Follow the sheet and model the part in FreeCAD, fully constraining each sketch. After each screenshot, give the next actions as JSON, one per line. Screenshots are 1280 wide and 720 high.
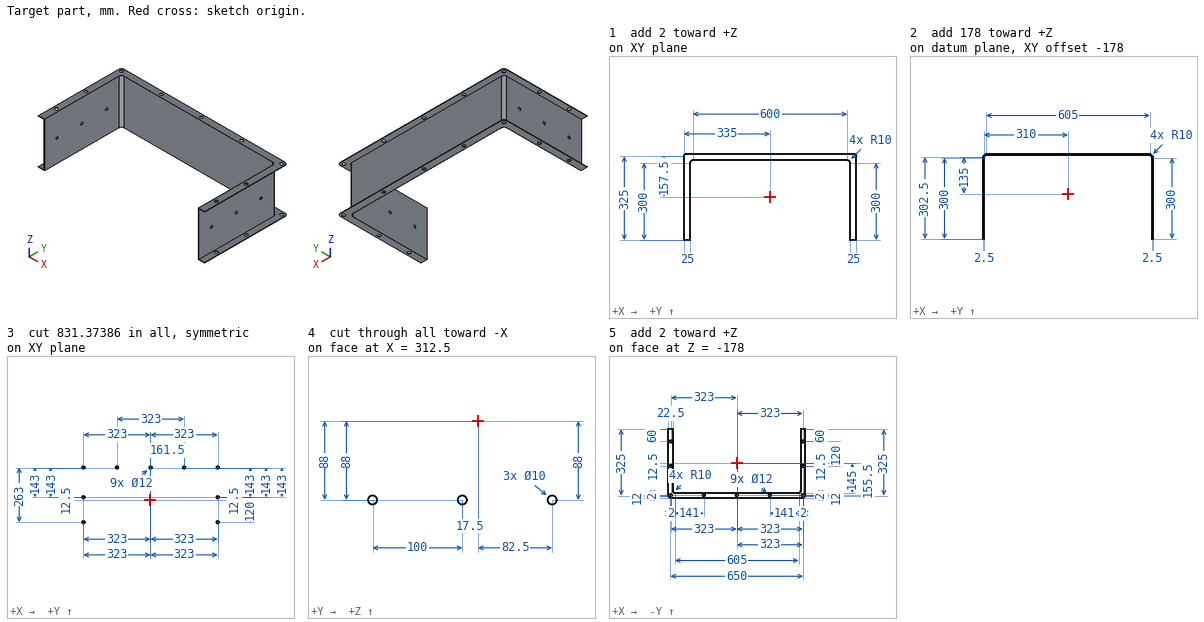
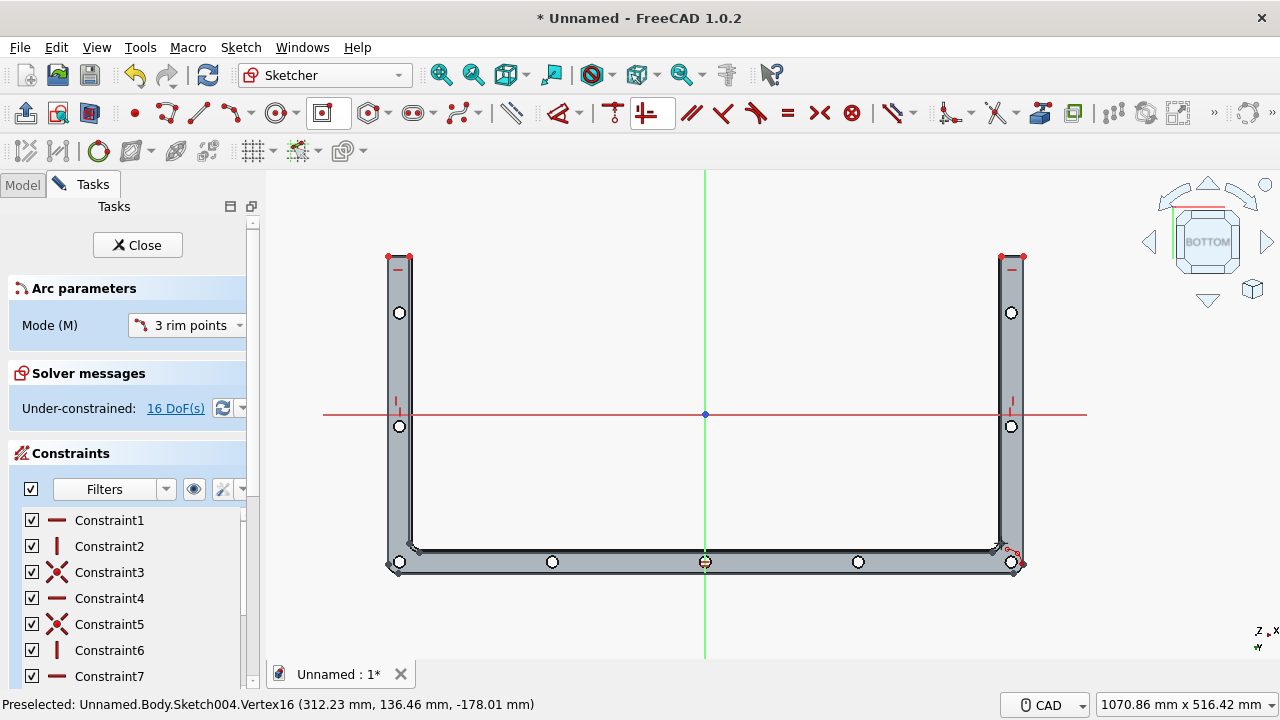
{"action": "left_click", "coordinate": [419, 553]}
{"action": "left_click", "coordinate": [409, 544]}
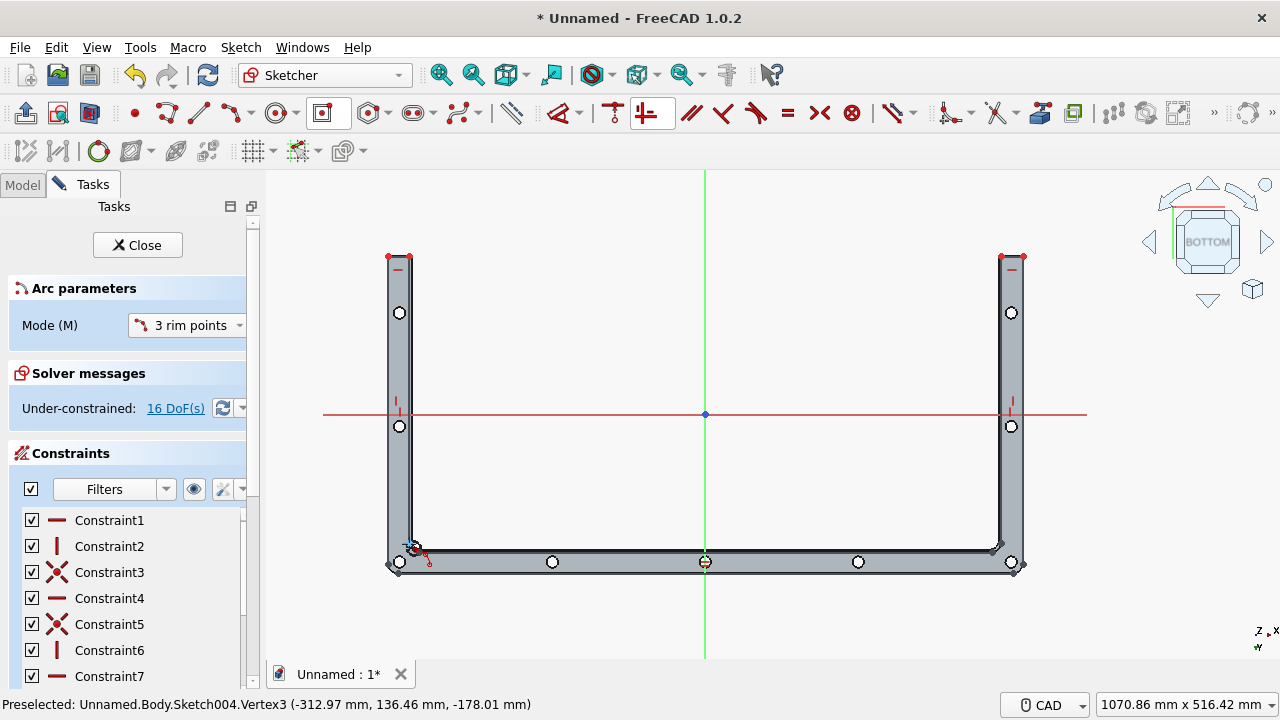
{"action": "scroll", "coordinate": [412, 549], "scroll_direction": "up", "scroll_amount": 9}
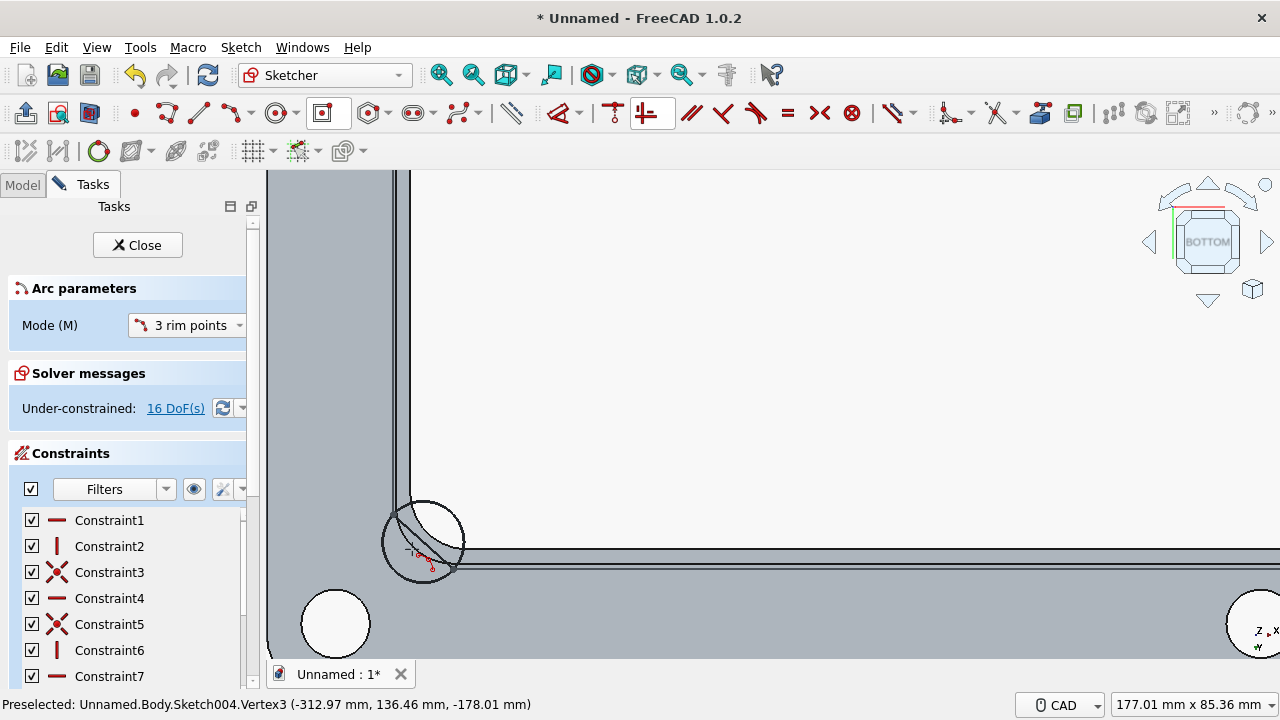
{"action": "left_click", "coordinate": [413, 547]}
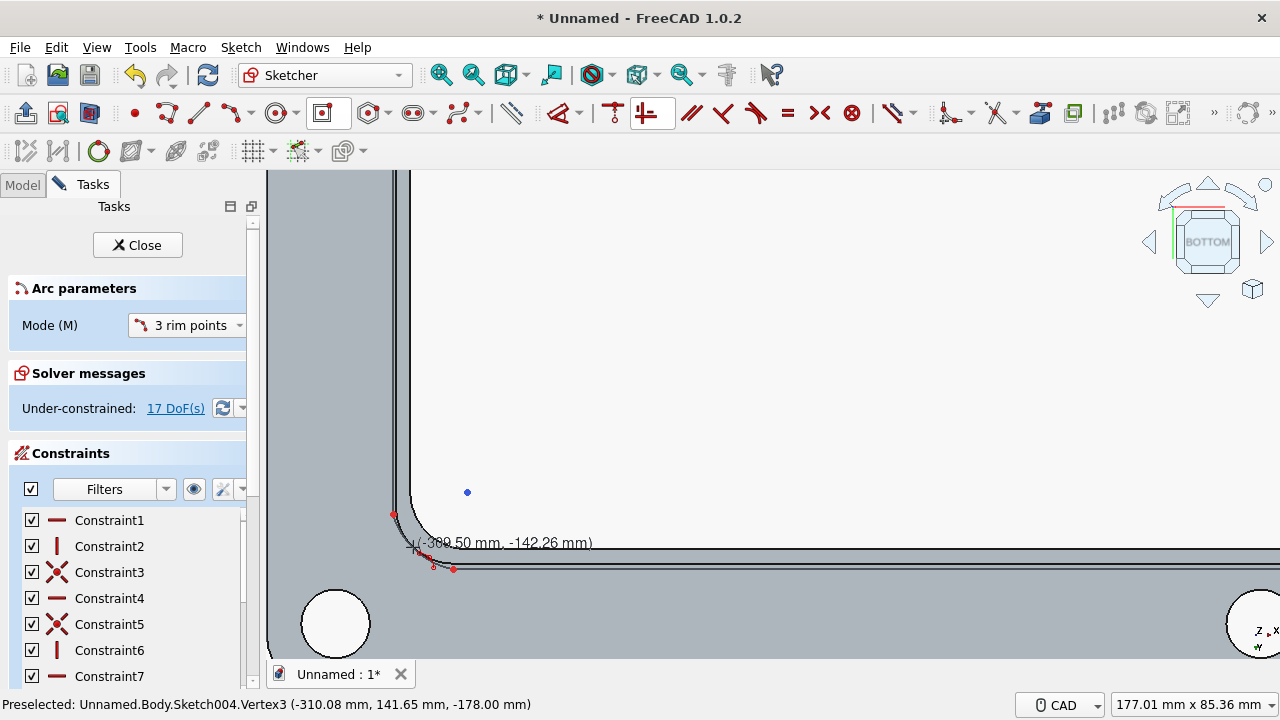
{"action": "scroll", "coordinate": [411, 549], "scroll_direction": "down", "scroll_amount": 9}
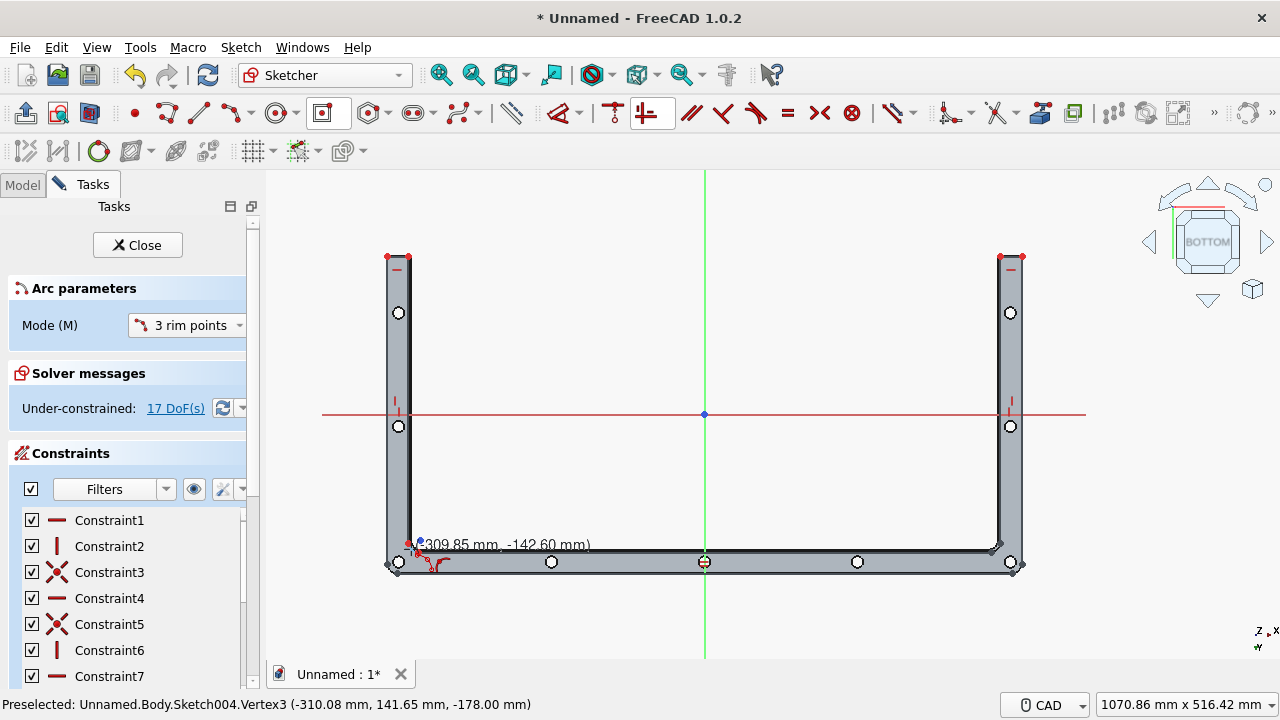
{"action": "left_click", "coordinate": [387, 565]}
{"action": "left_click", "coordinate": [397, 574]}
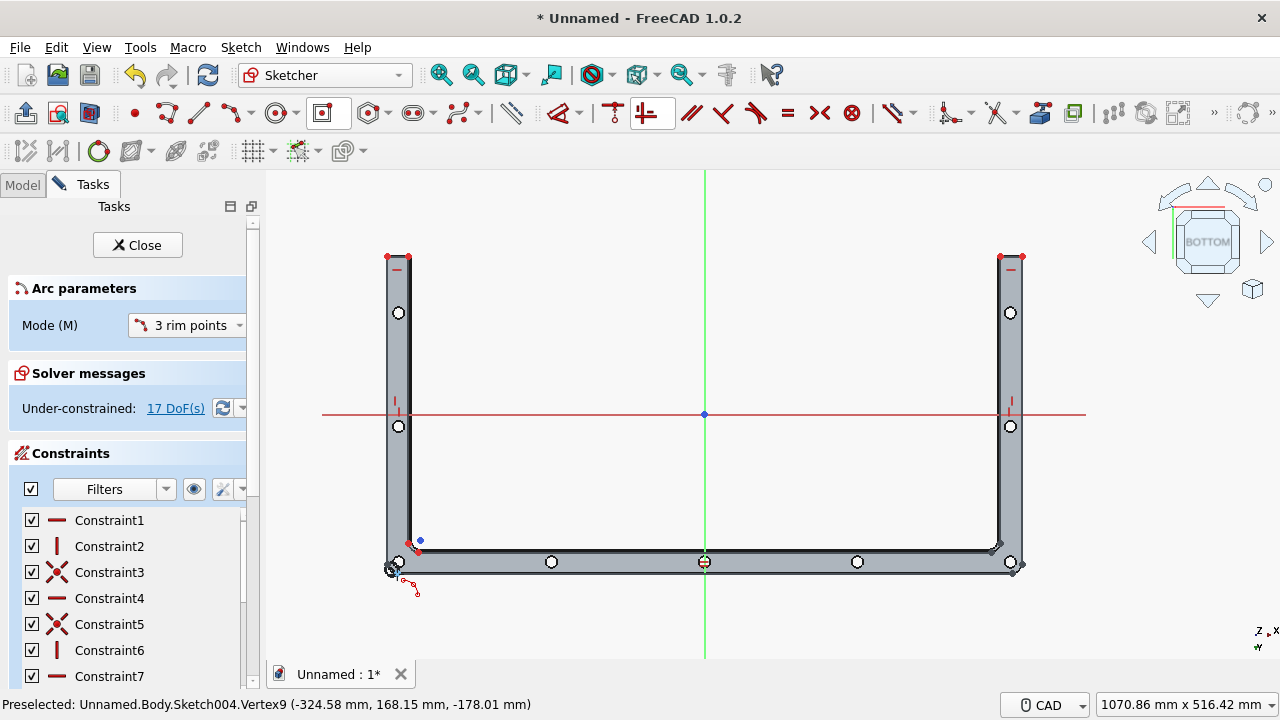
{"action": "scroll", "coordinate": [390, 571], "scroll_direction": "up", "scroll_amount": 9}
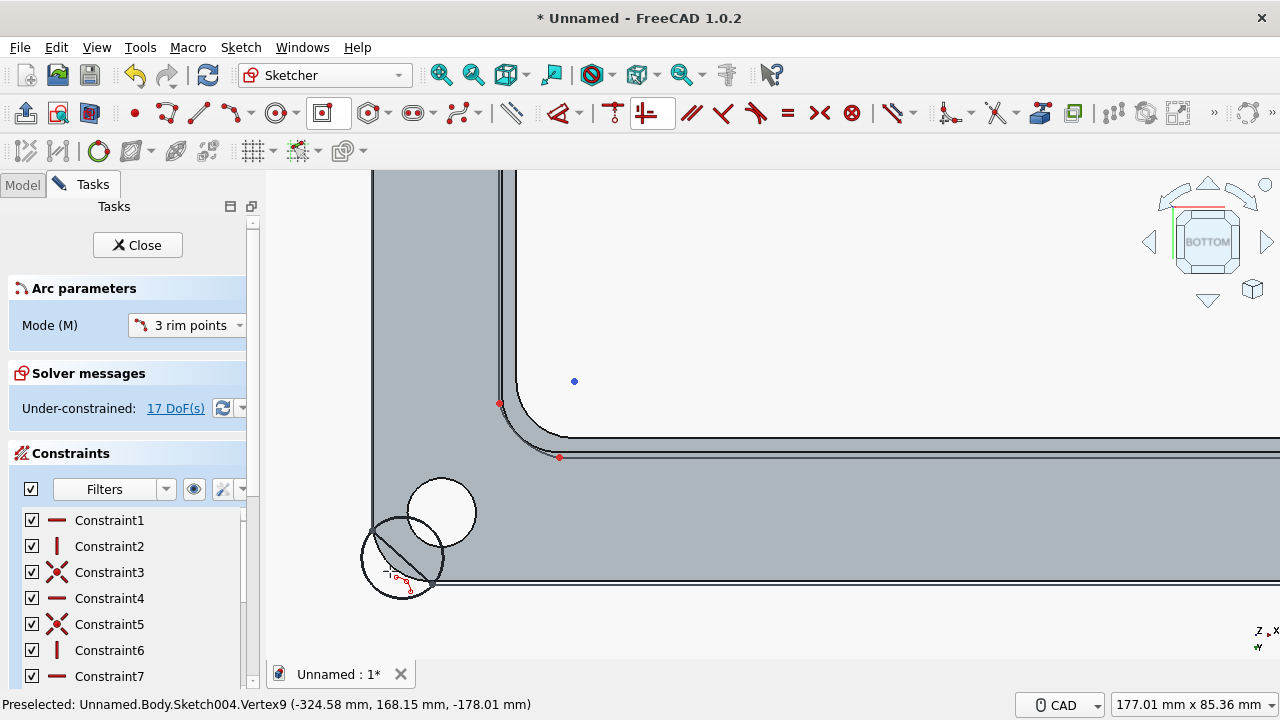
{"action": "left_click", "coordinate": [390, 565]}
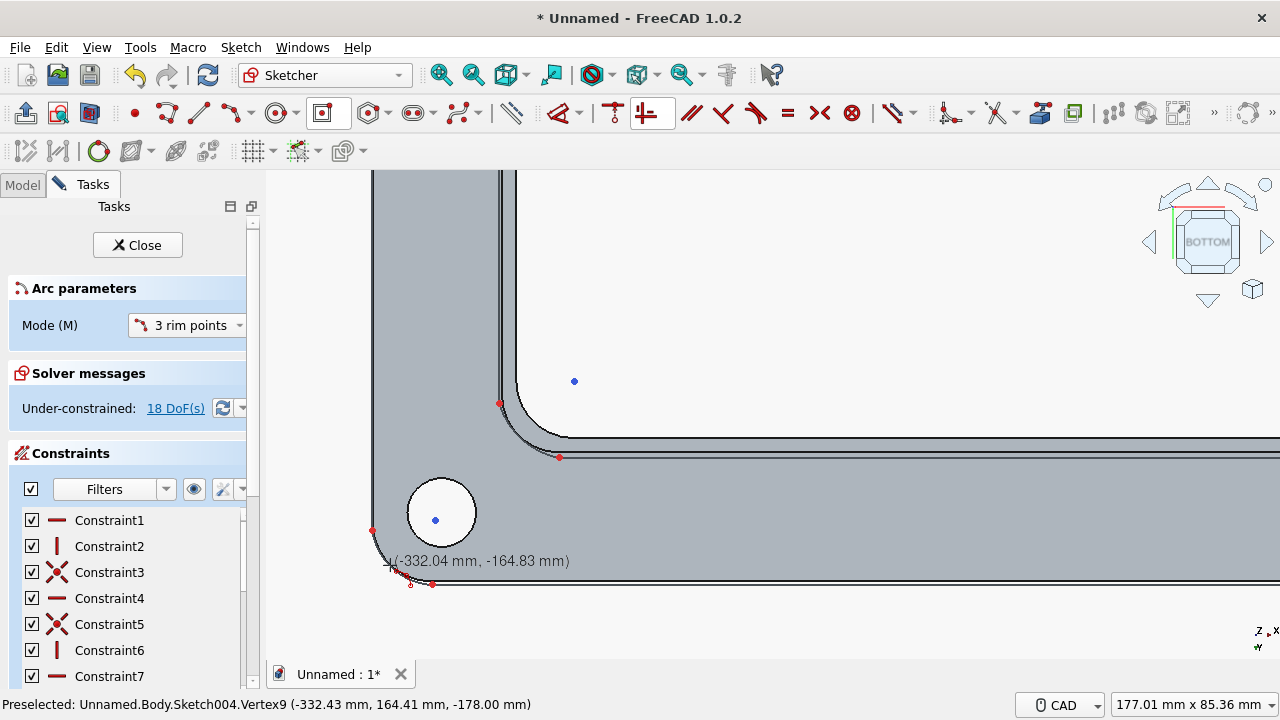
{"action": "scroll", "coordinate": [390, 571], "scroll_direction": "down", "scroll_amount": 9}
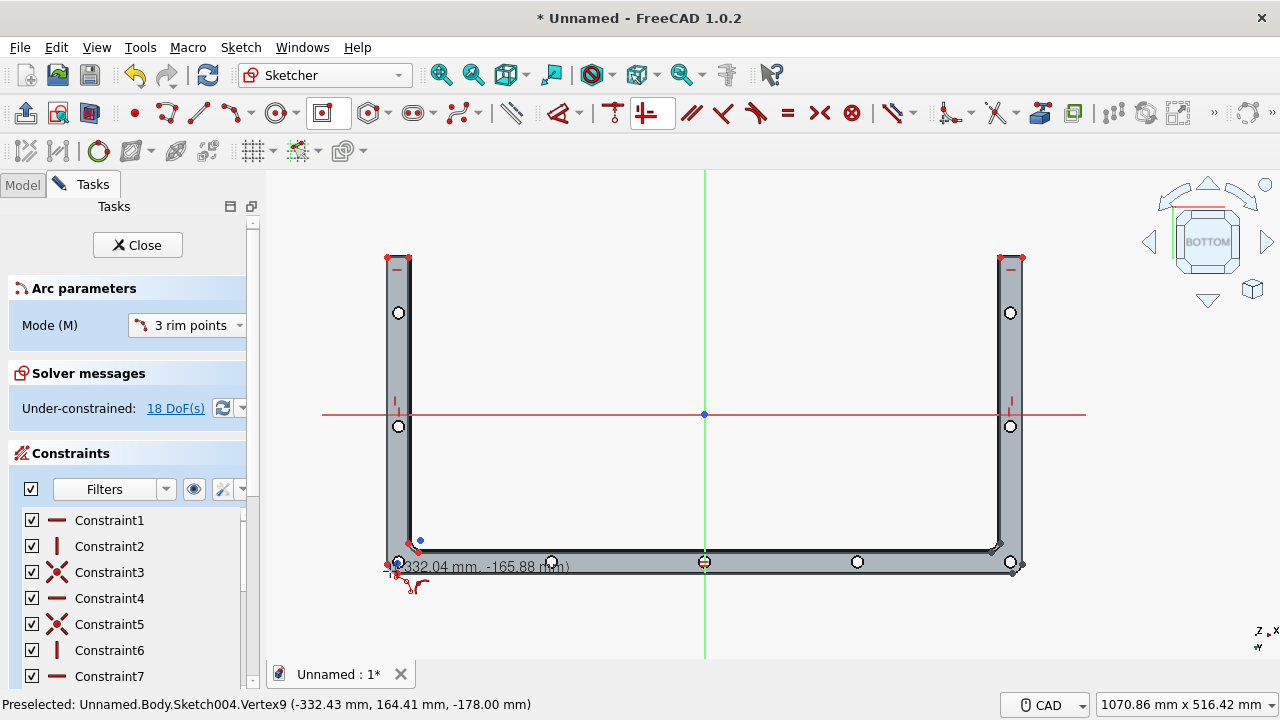
{"action": "left_click", "coordinate": [1012, 574]}
{"action": "left_click", "coordinate": [1022, 565]}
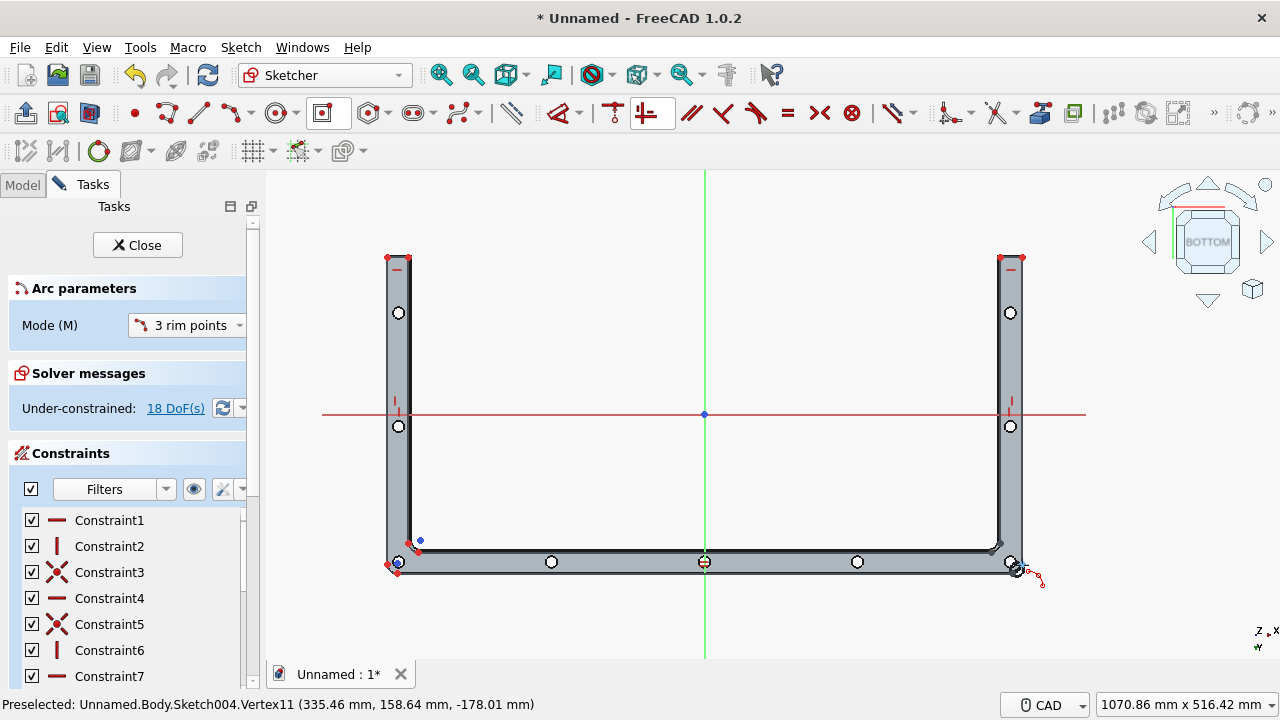
{"action": "scroll", "coordinate": [1019, 571], "scroll_direction": "up", "scroll_amount": 9}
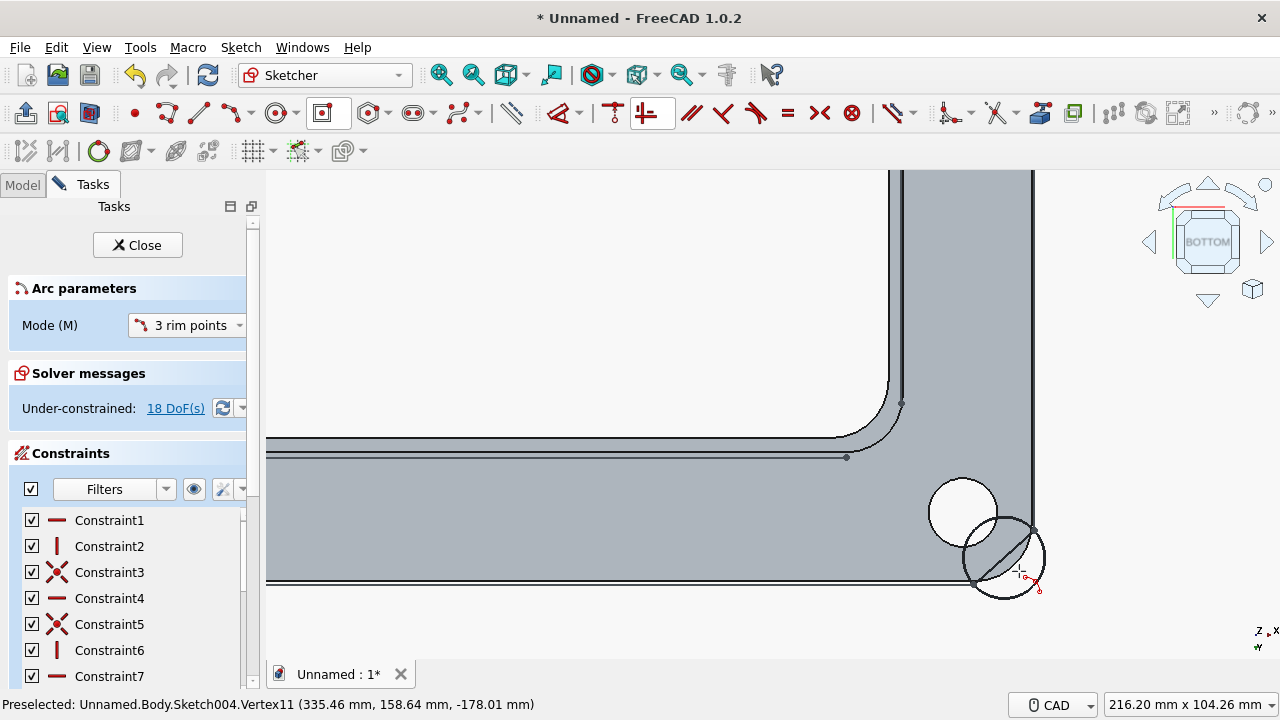
{"action": "left_click", "coordinate": [1015, 565]}